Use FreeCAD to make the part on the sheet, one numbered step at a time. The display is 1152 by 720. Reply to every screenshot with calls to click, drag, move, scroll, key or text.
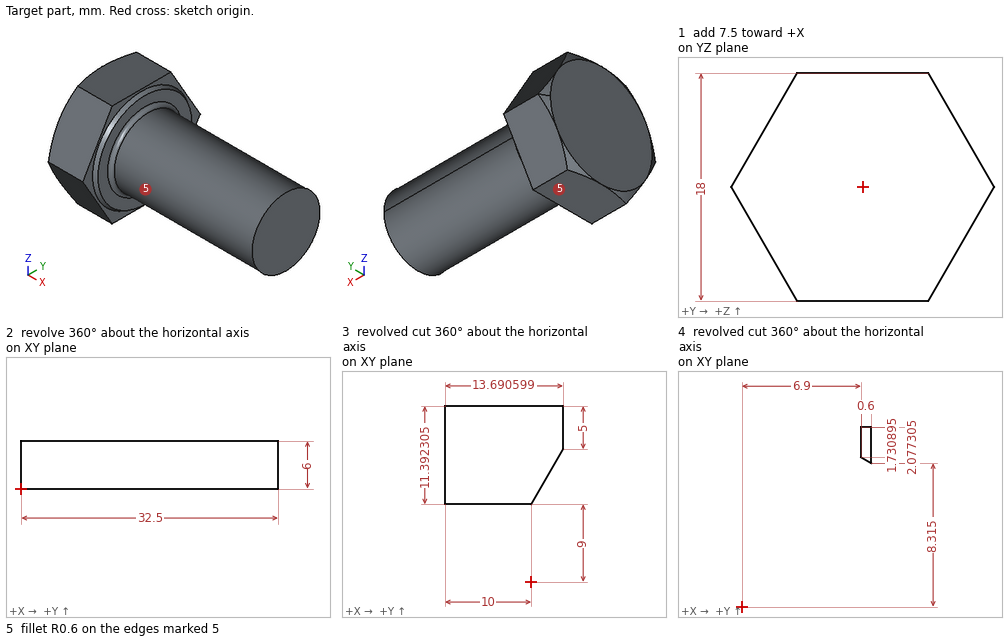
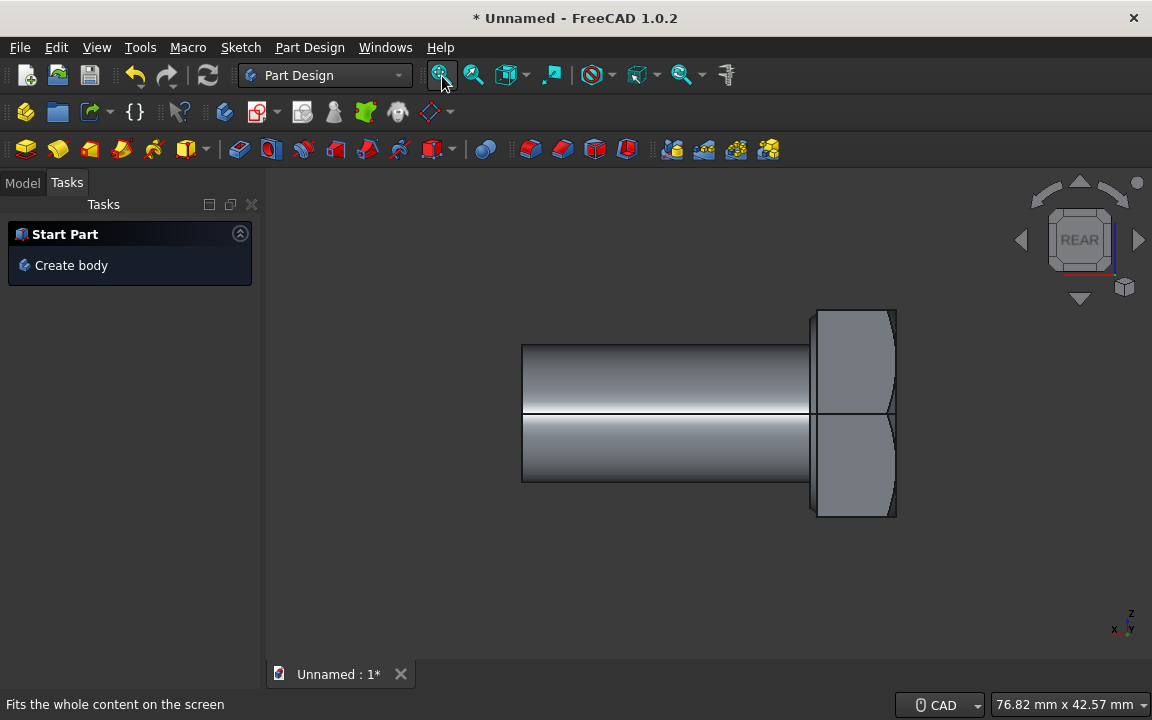
key(6)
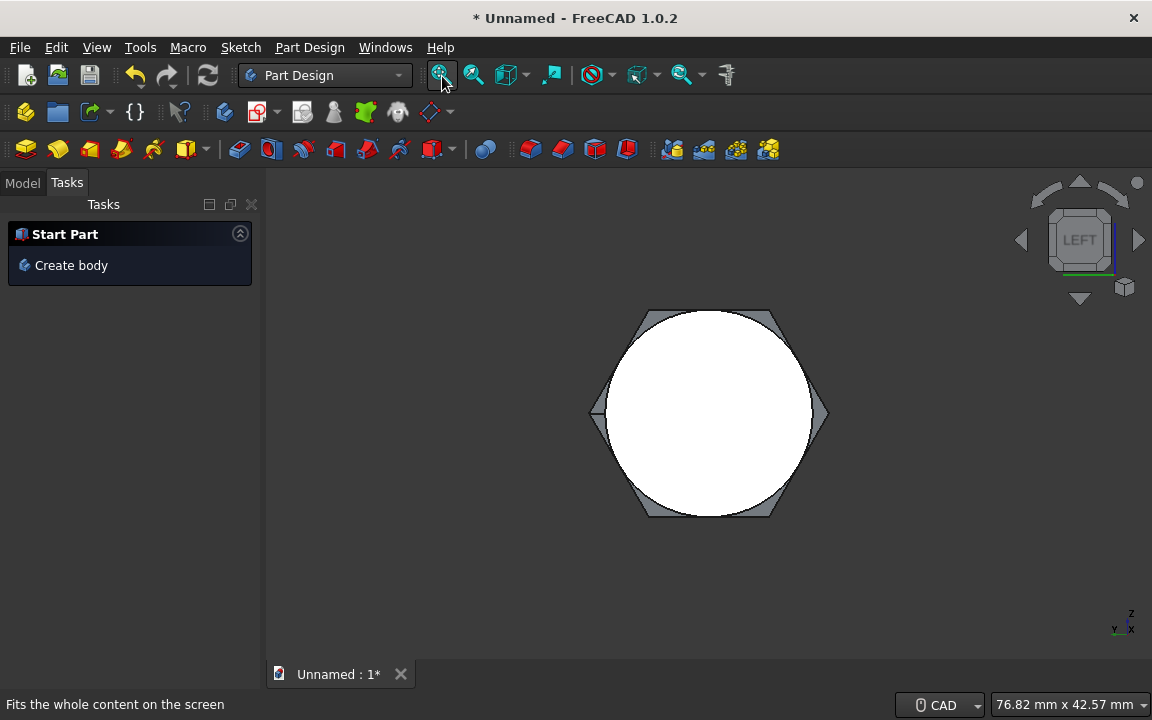
click(442, 76)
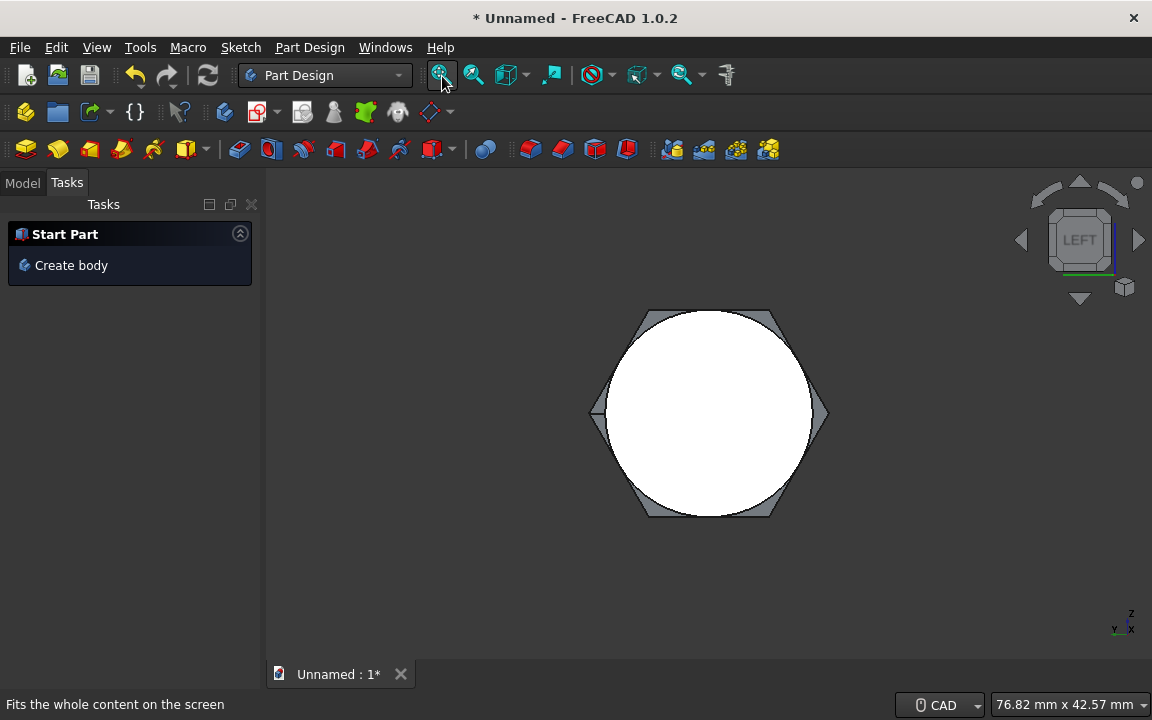
key(v)
key(3)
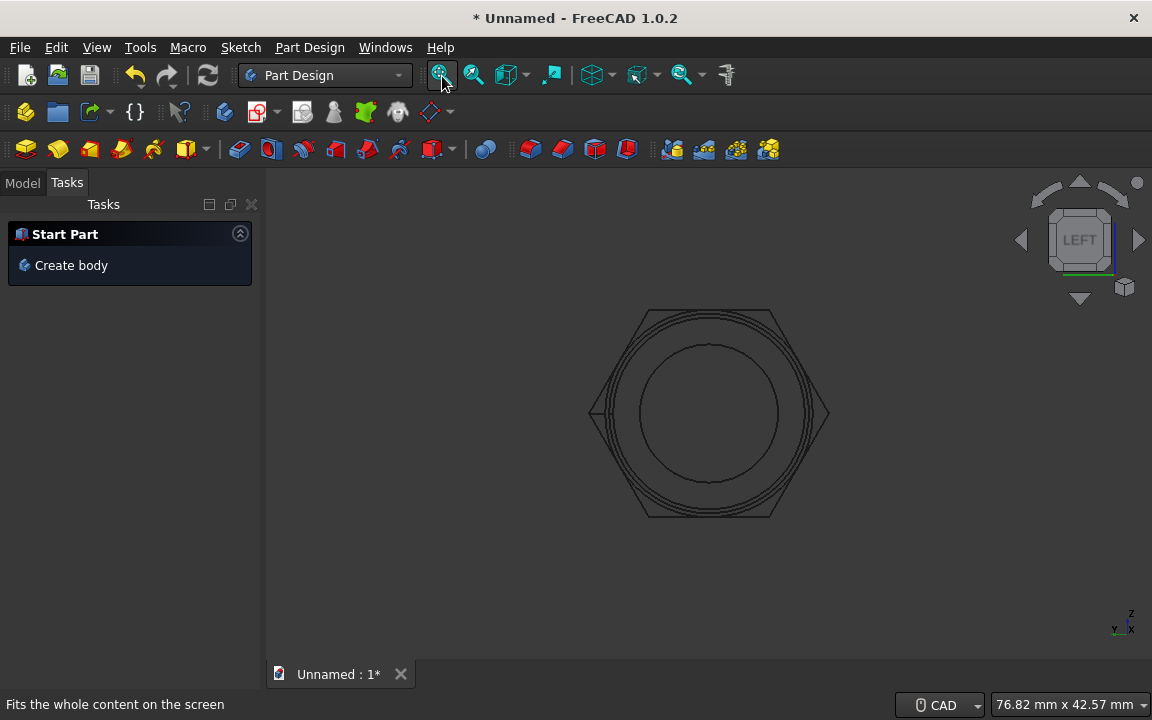
key(0)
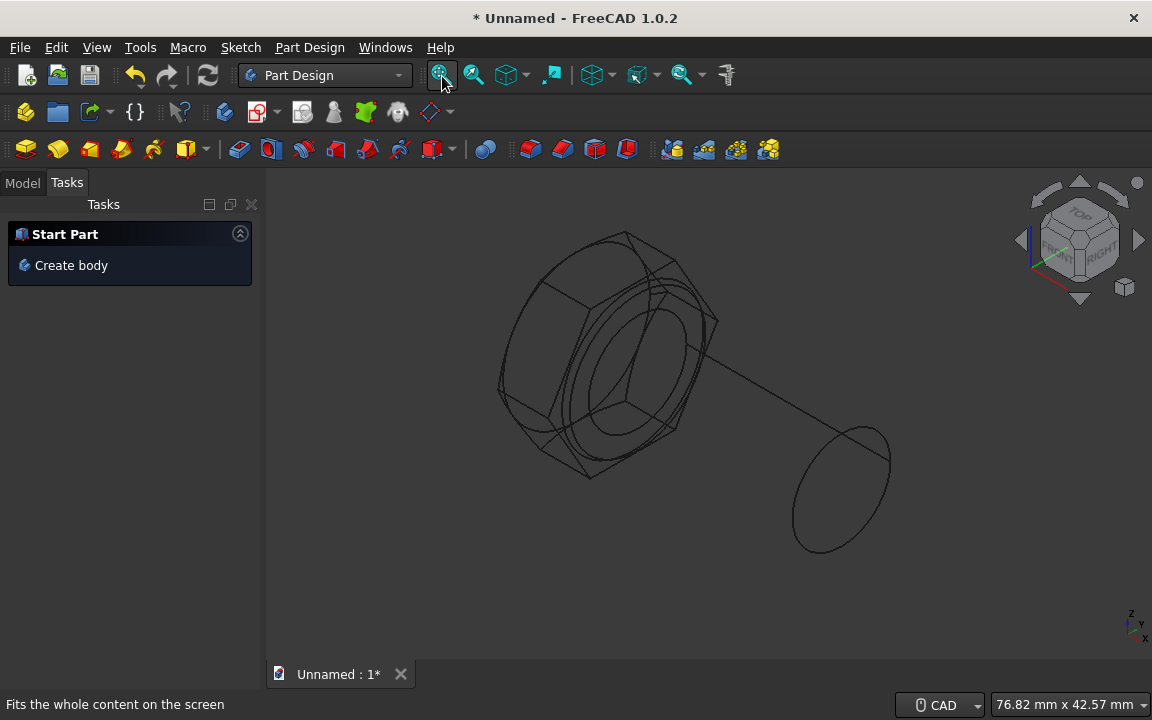
click(589, 400)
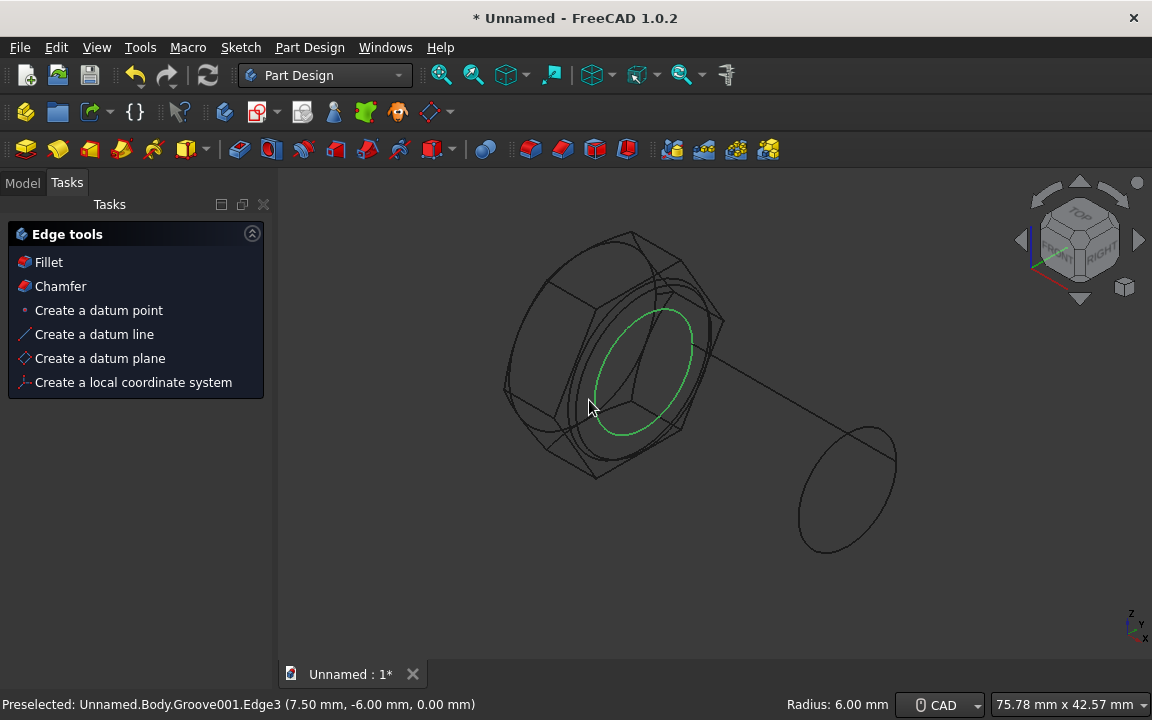
key(v)
key(1)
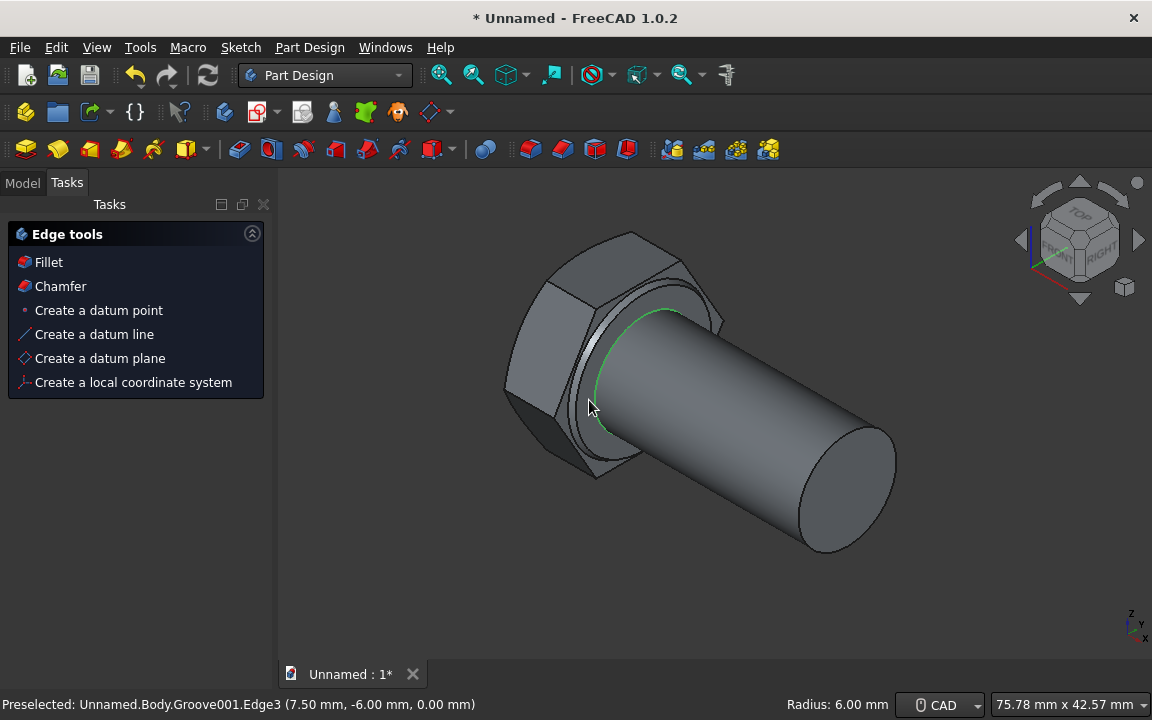
click(532, 150)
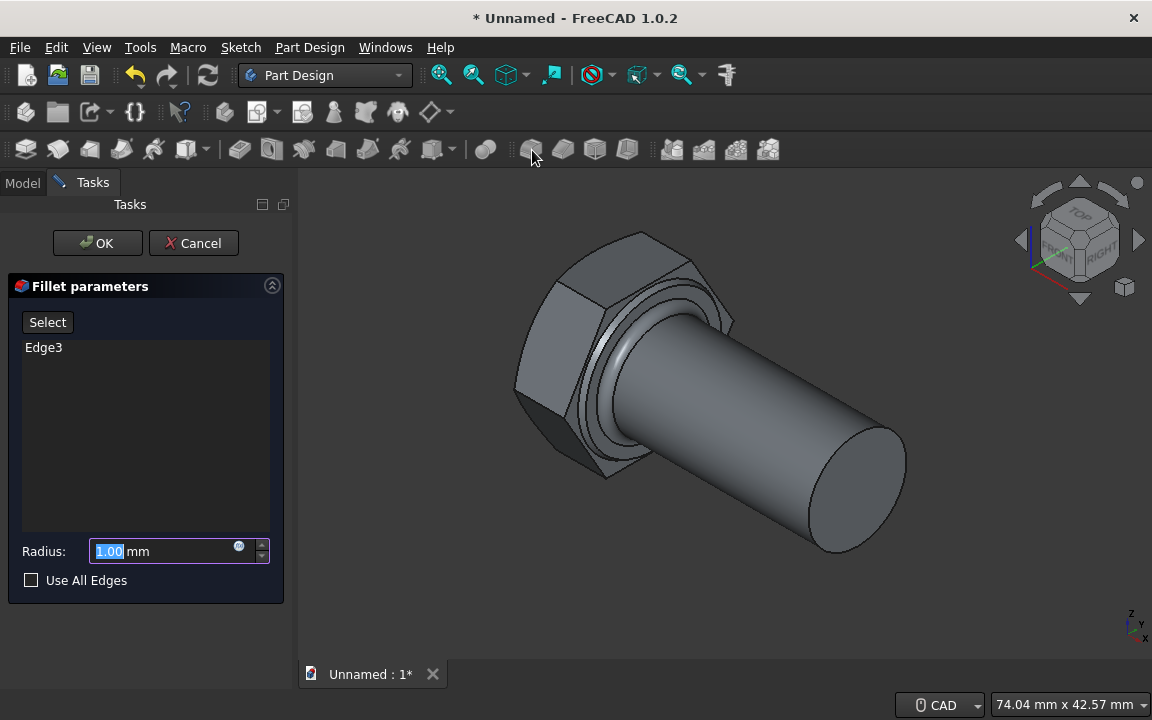
text(0.6)
key(Tab)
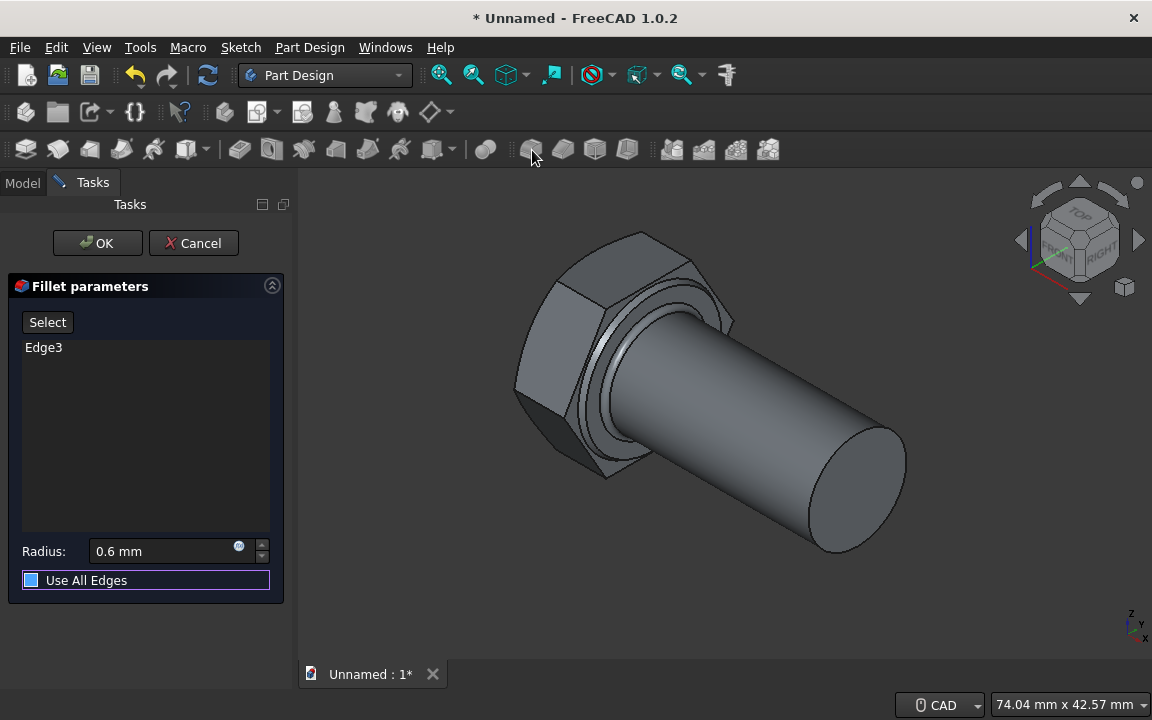
click(98, 243)